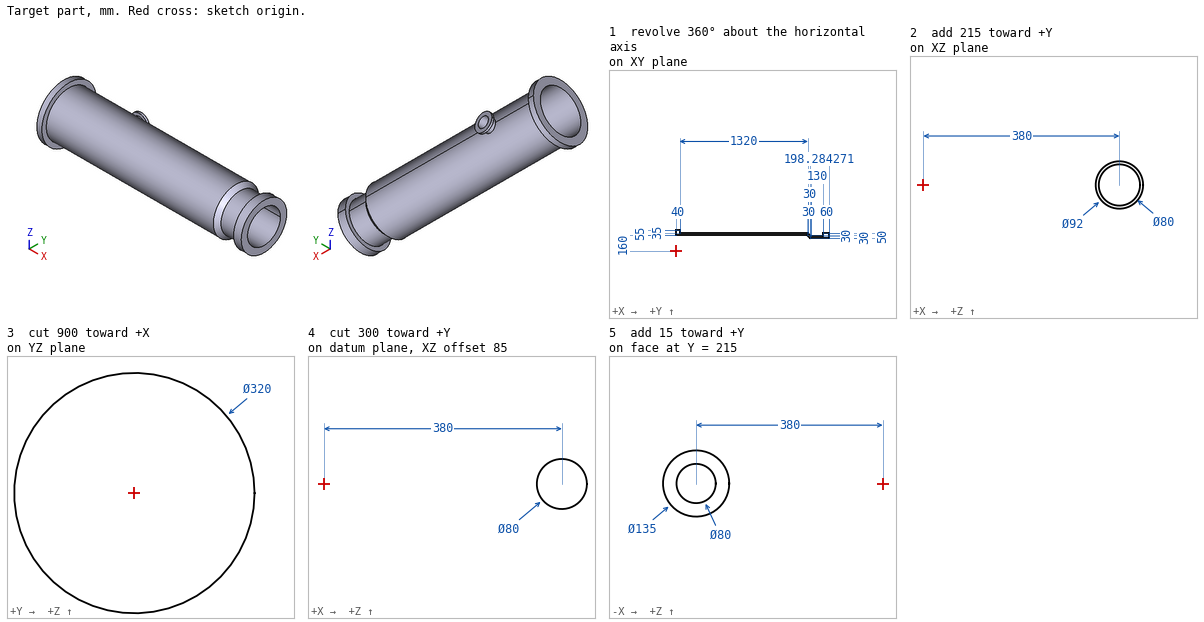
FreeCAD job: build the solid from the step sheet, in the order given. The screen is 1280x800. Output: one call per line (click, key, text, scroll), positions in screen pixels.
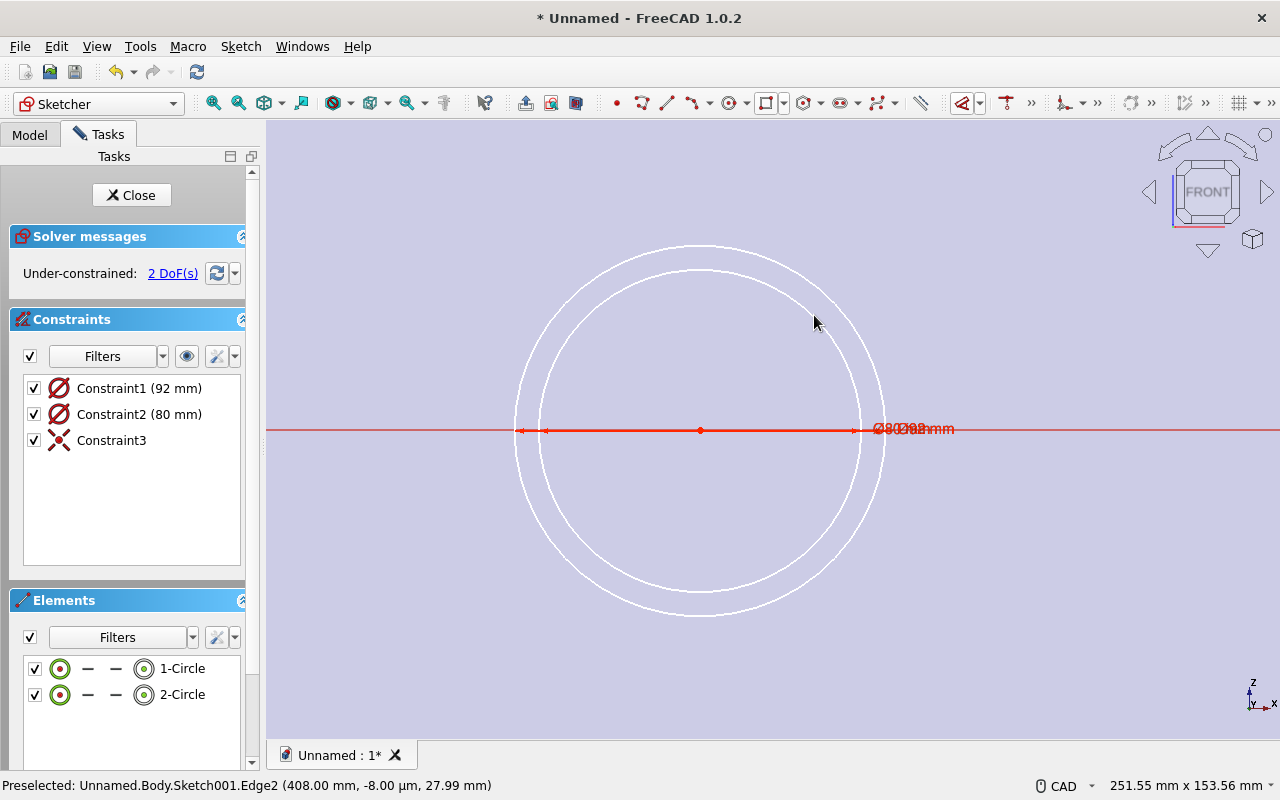
click(700, 431)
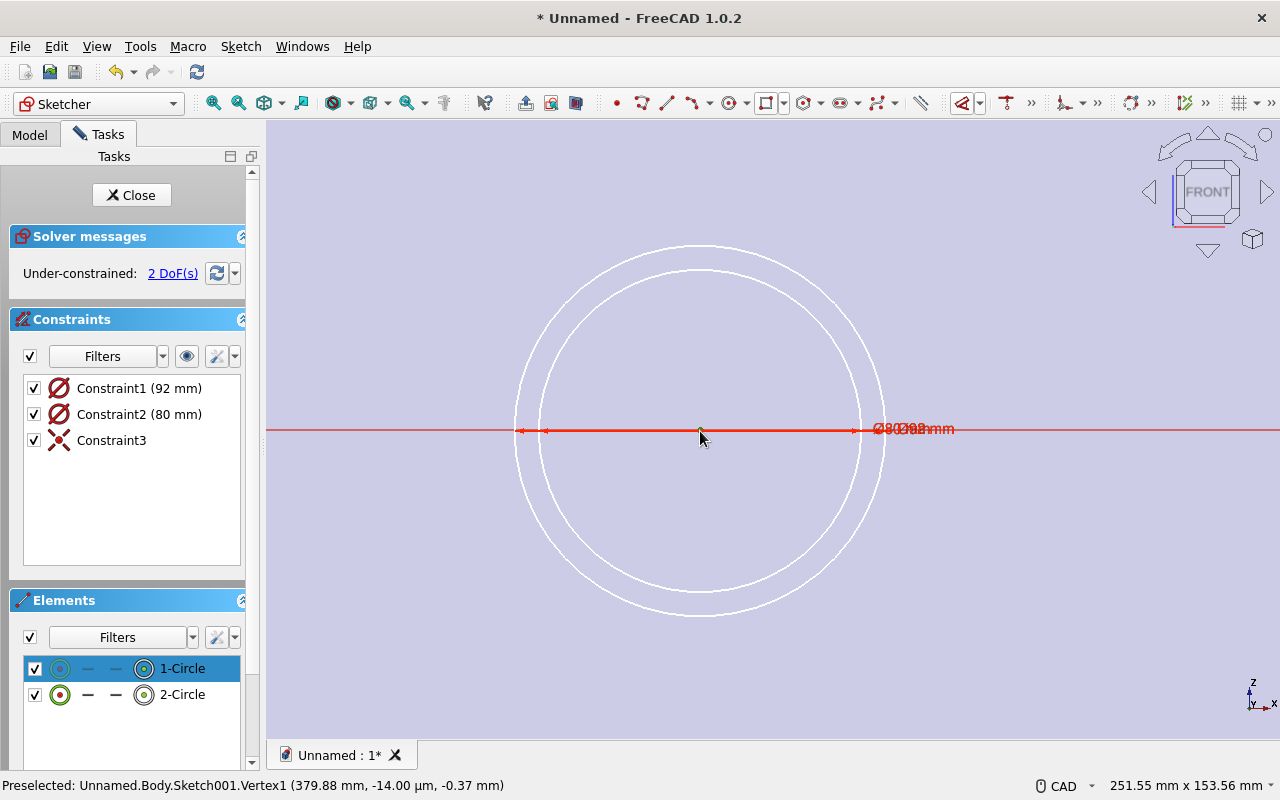
click(353, 430)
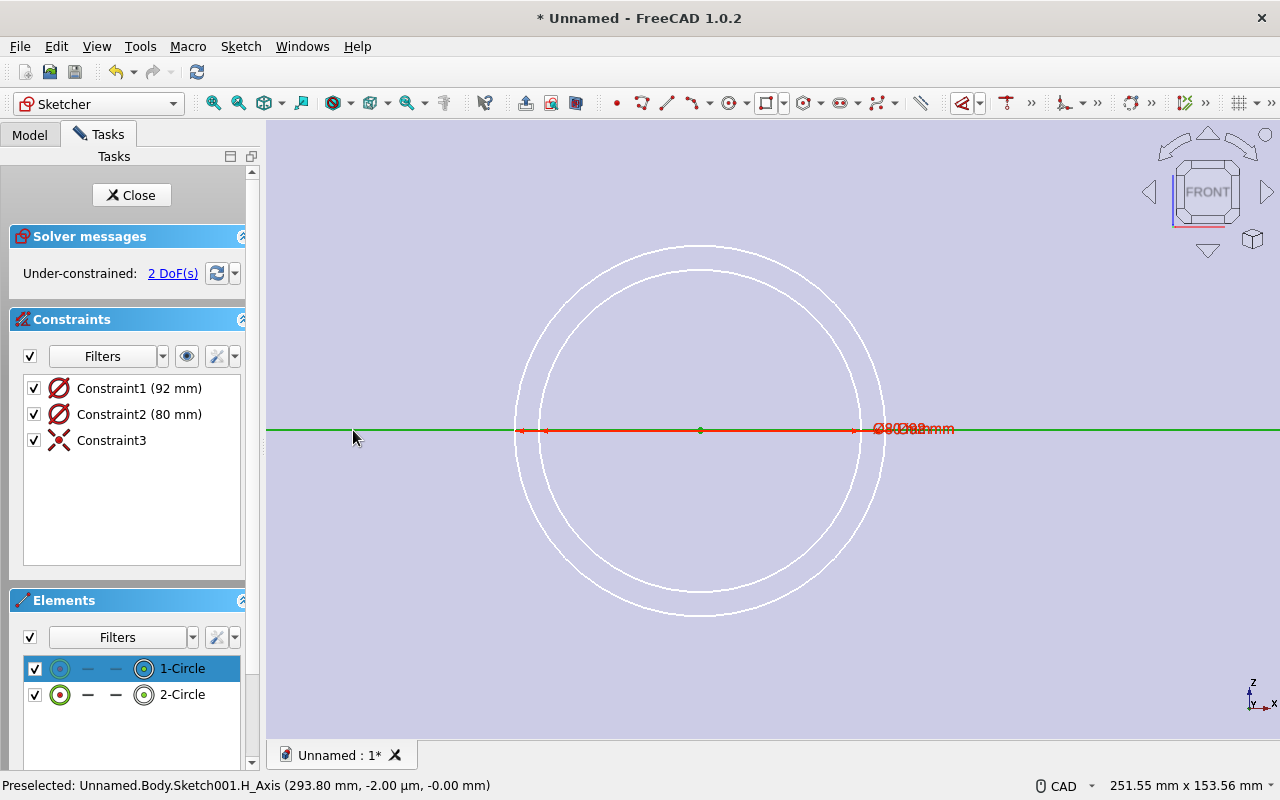
key(c)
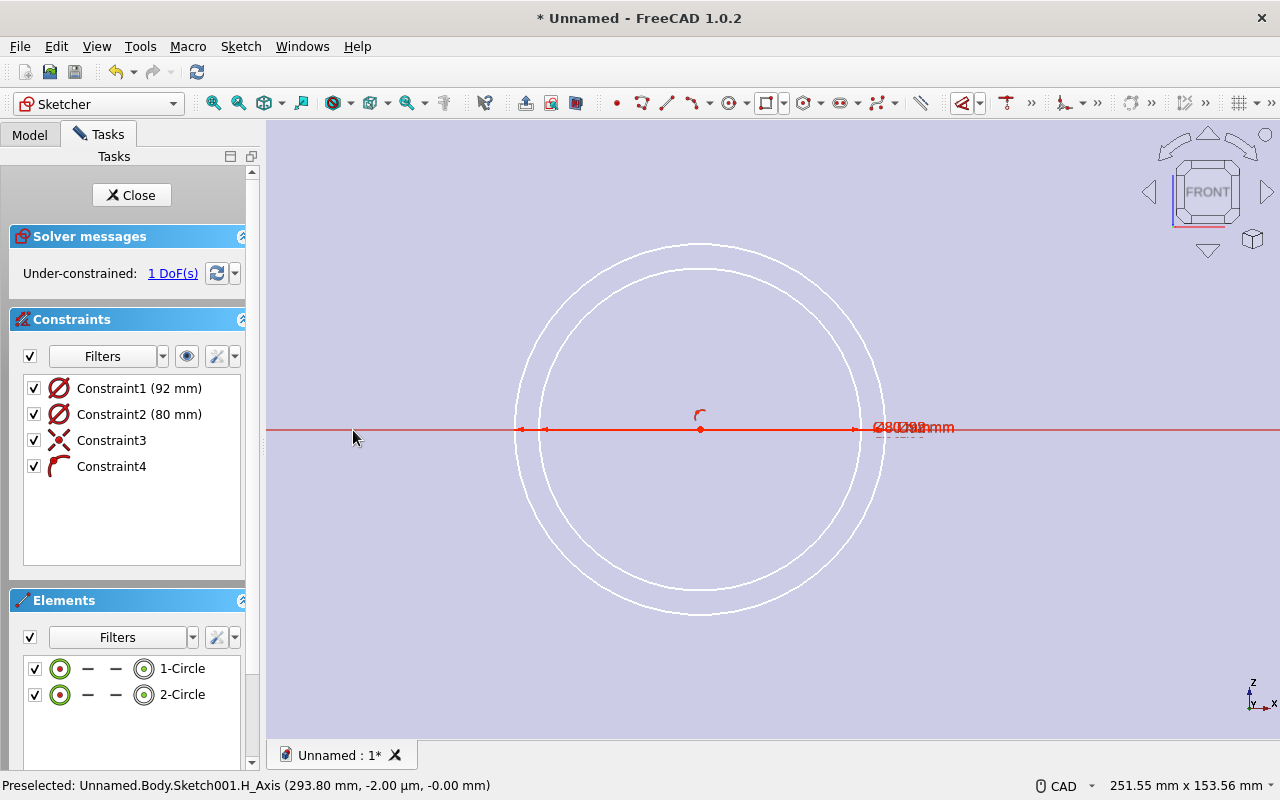
click(700, 430)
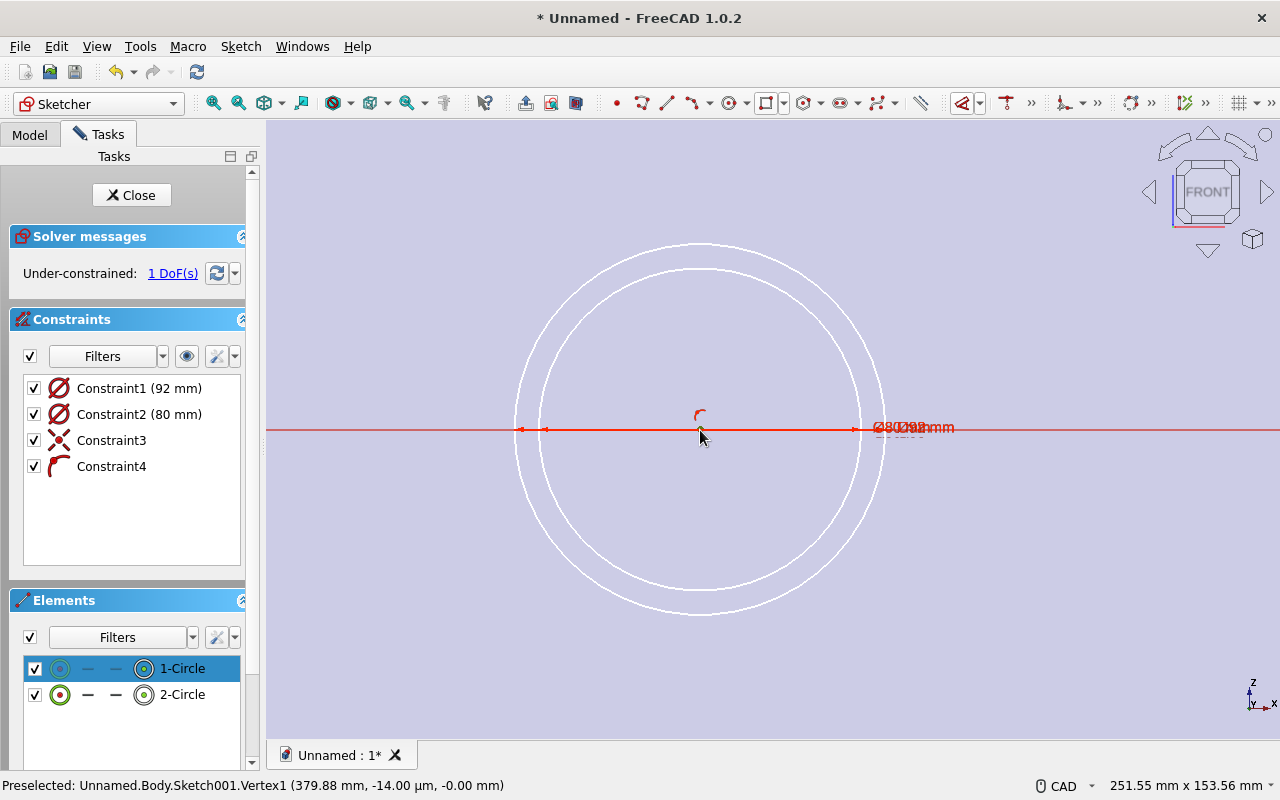
key(l)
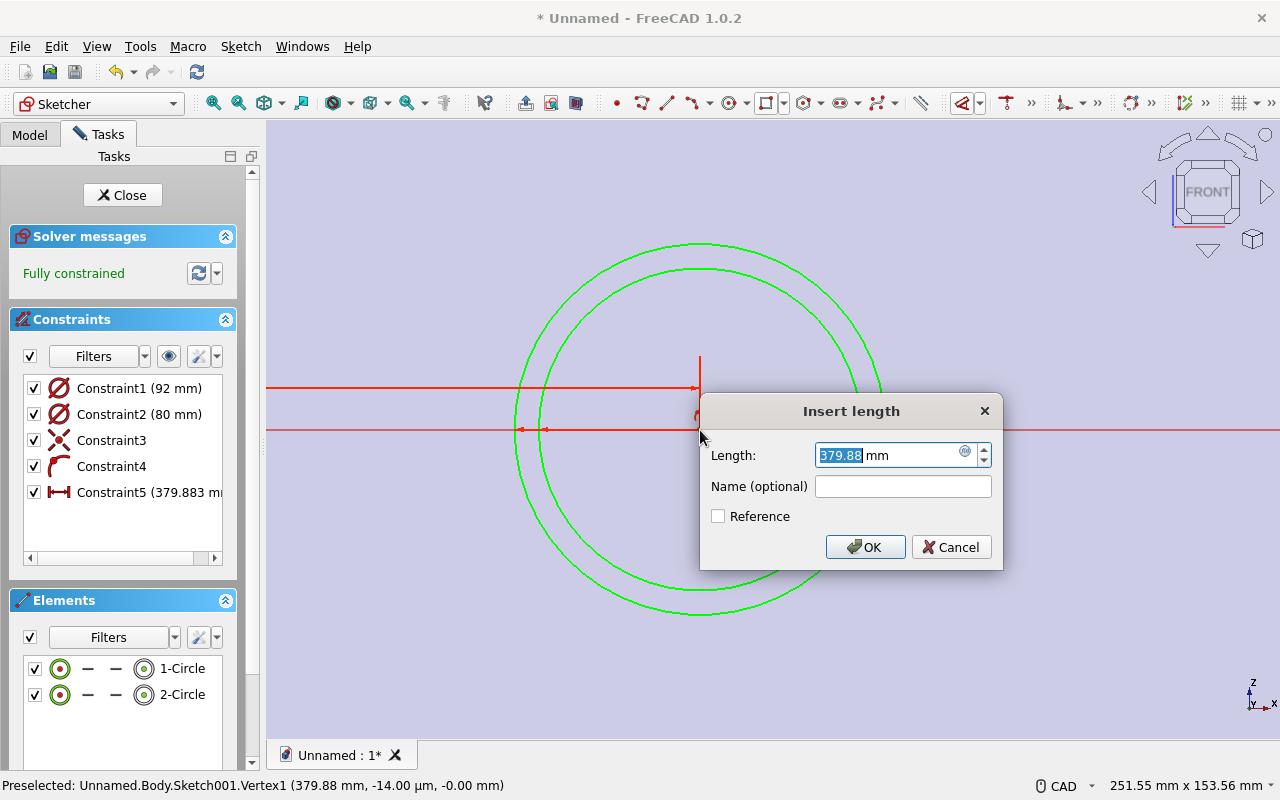
text(380)
key(Return)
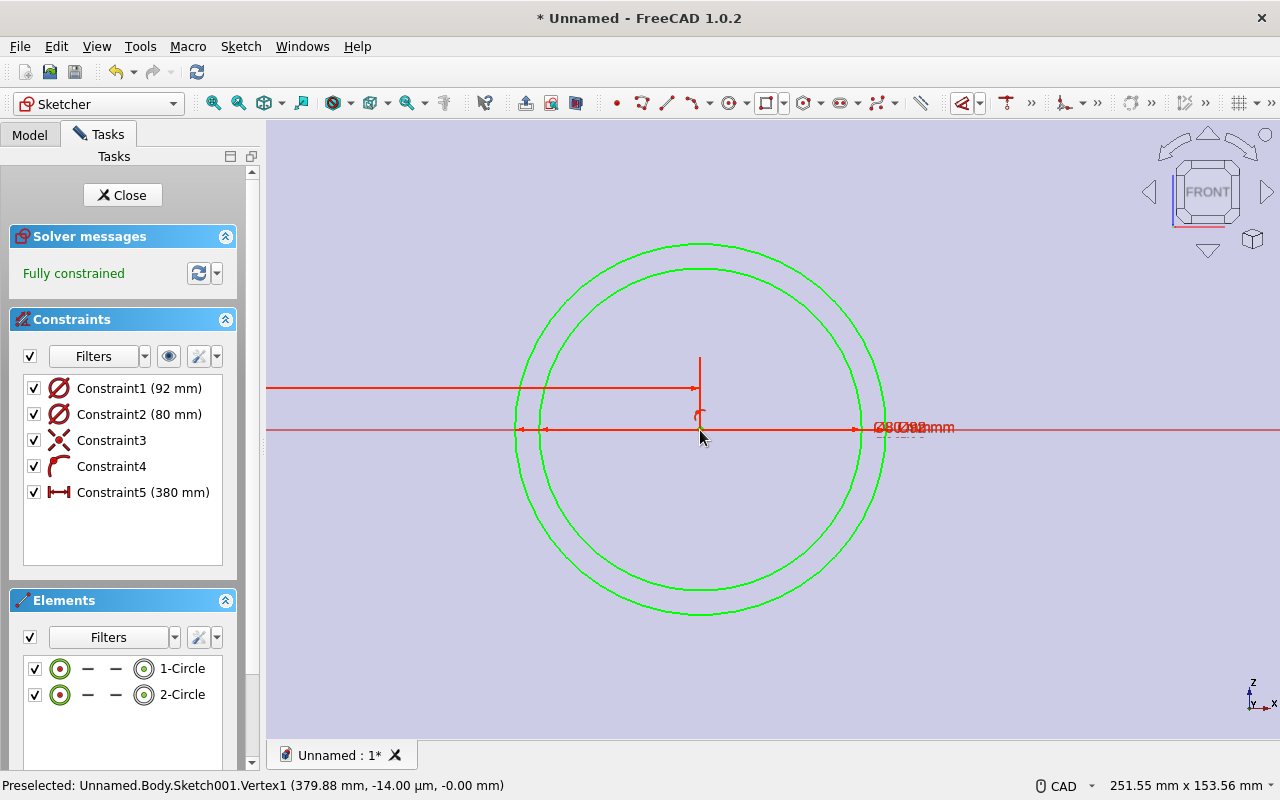
click(123, 195)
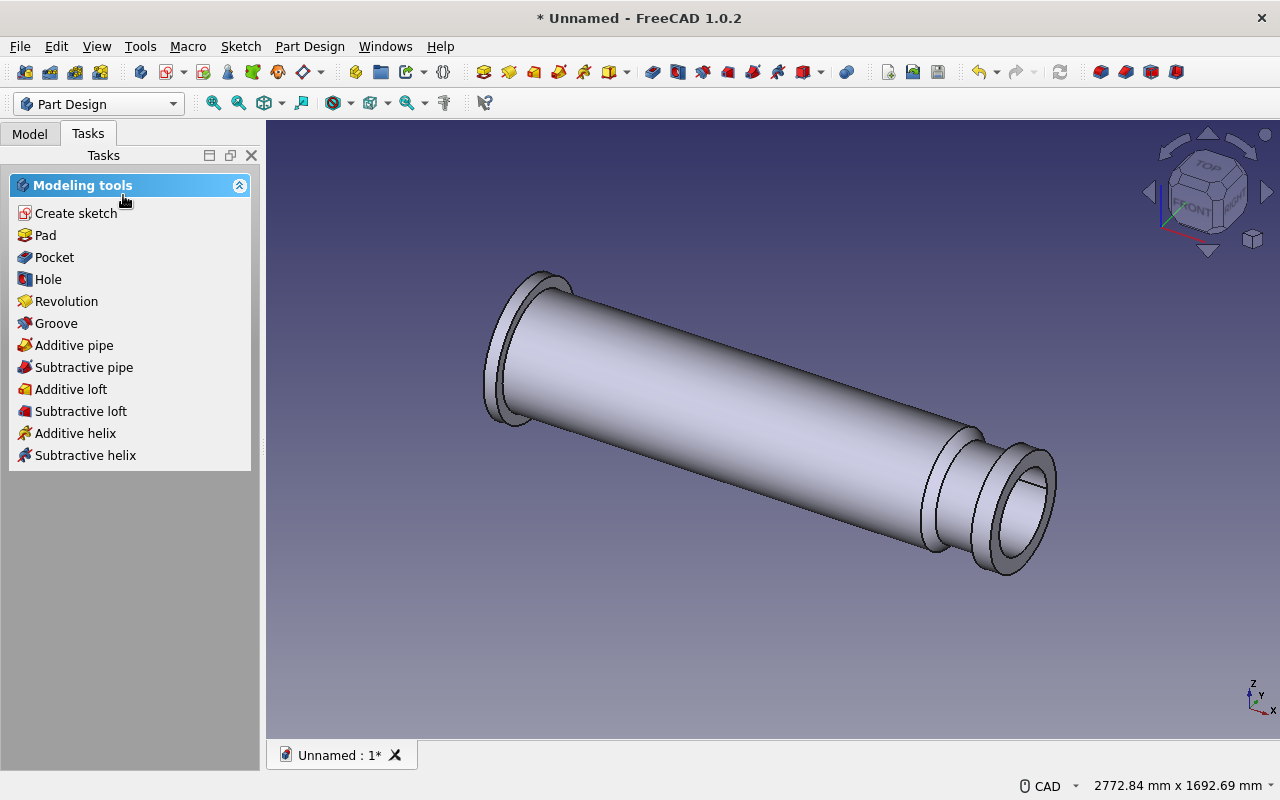
click(484, 72)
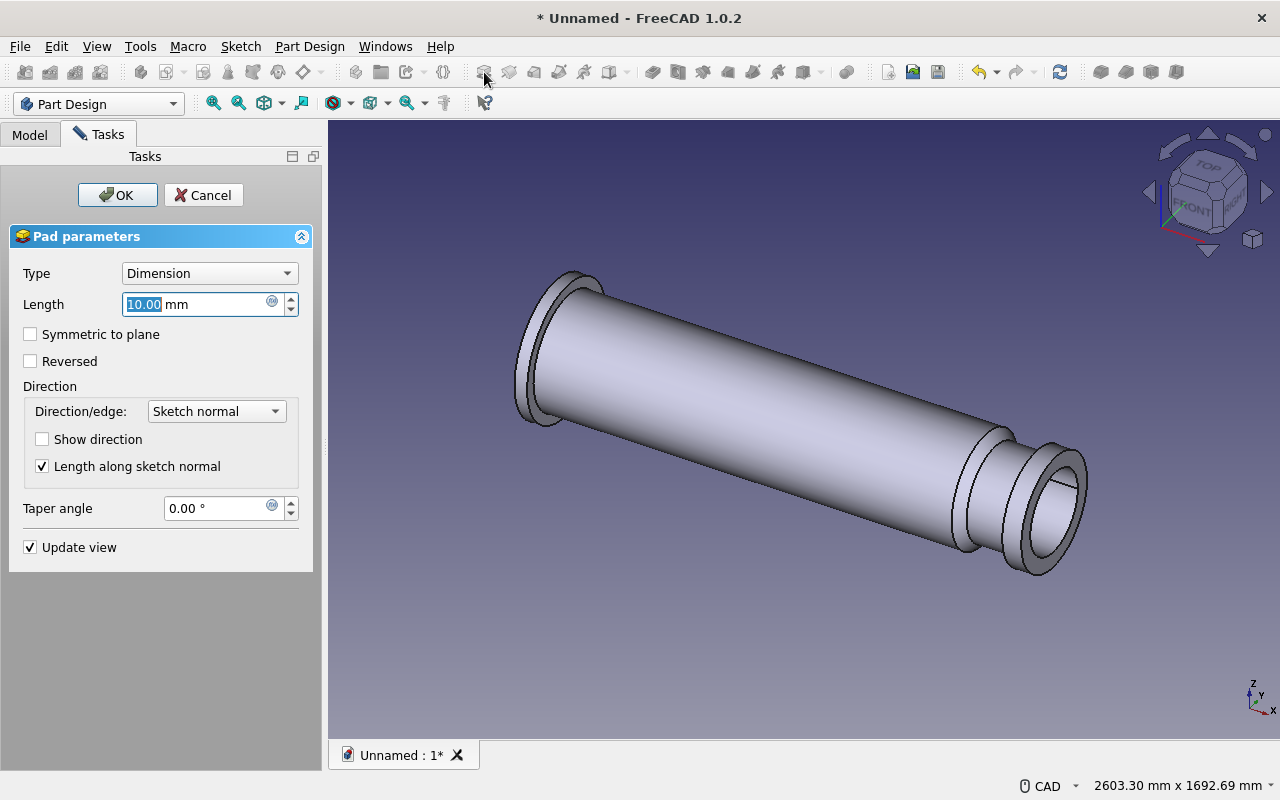
text(215)
key(Tab)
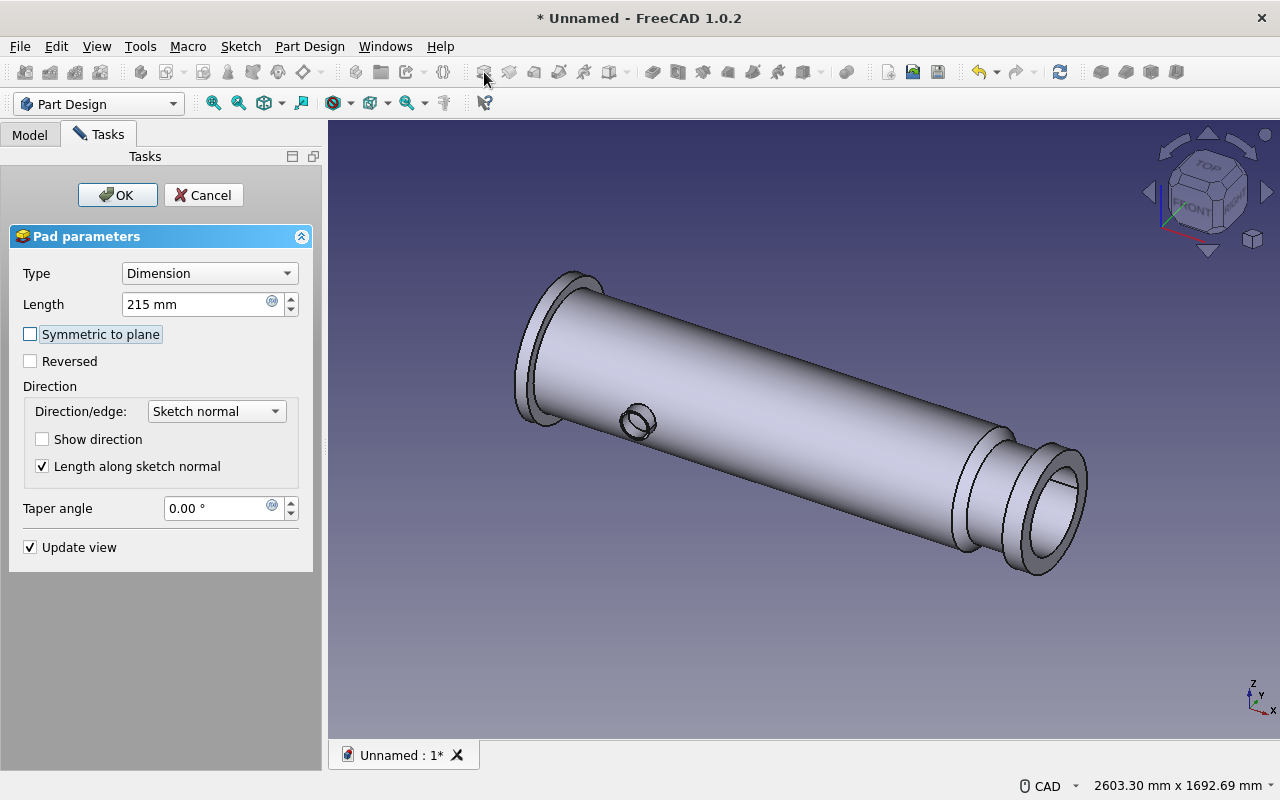
click(31, 361)